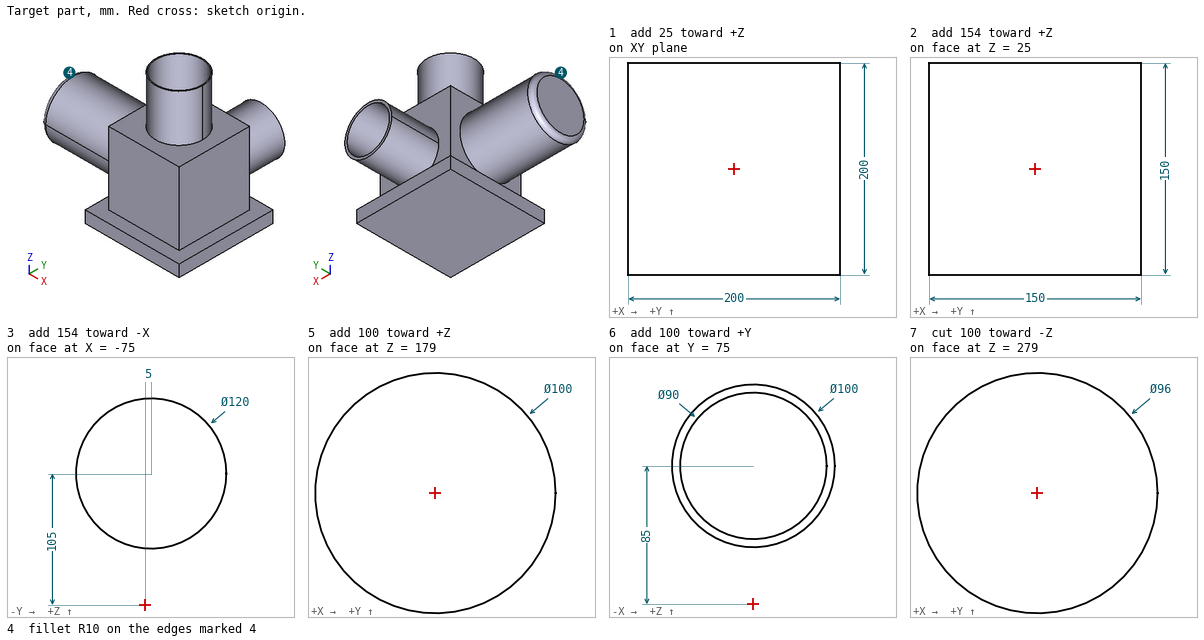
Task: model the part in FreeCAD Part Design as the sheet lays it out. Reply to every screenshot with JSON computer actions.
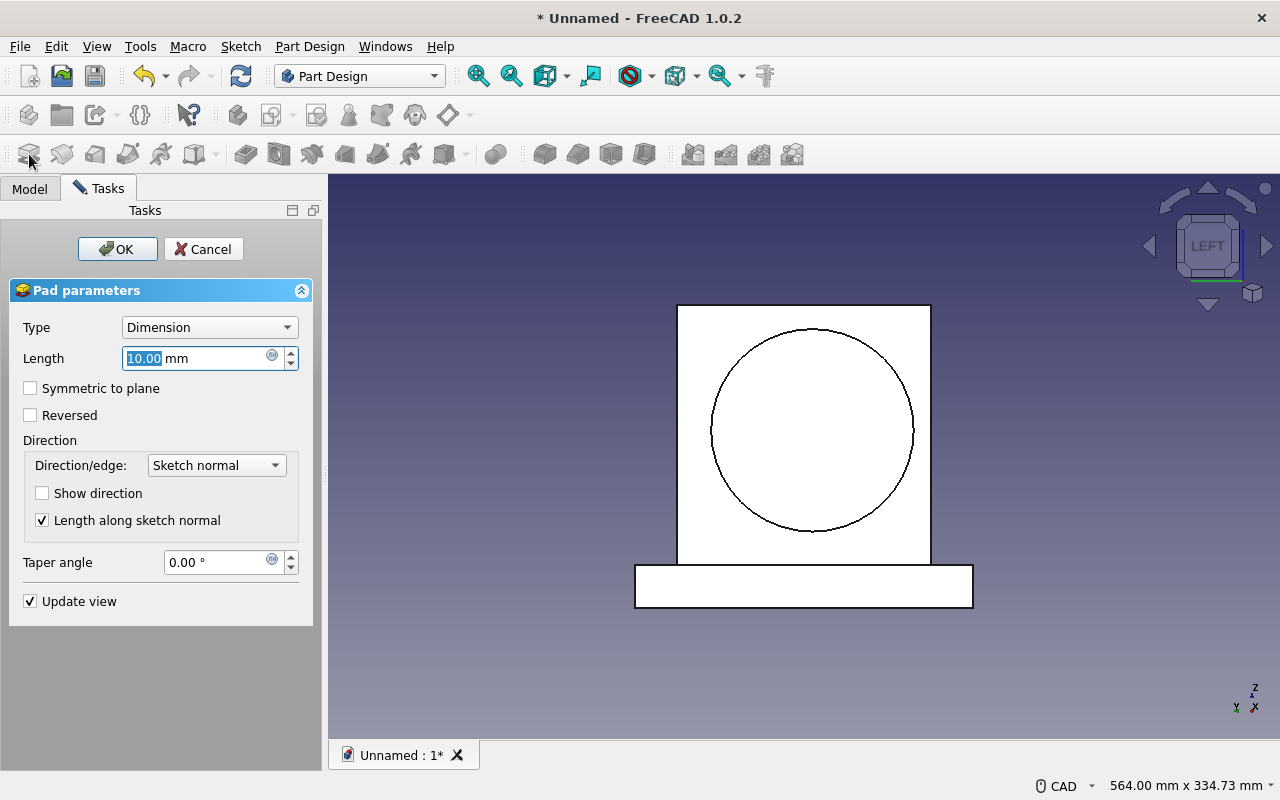
{"action": "type", "text": "154"}
{"action": "key", "text": "Tab"}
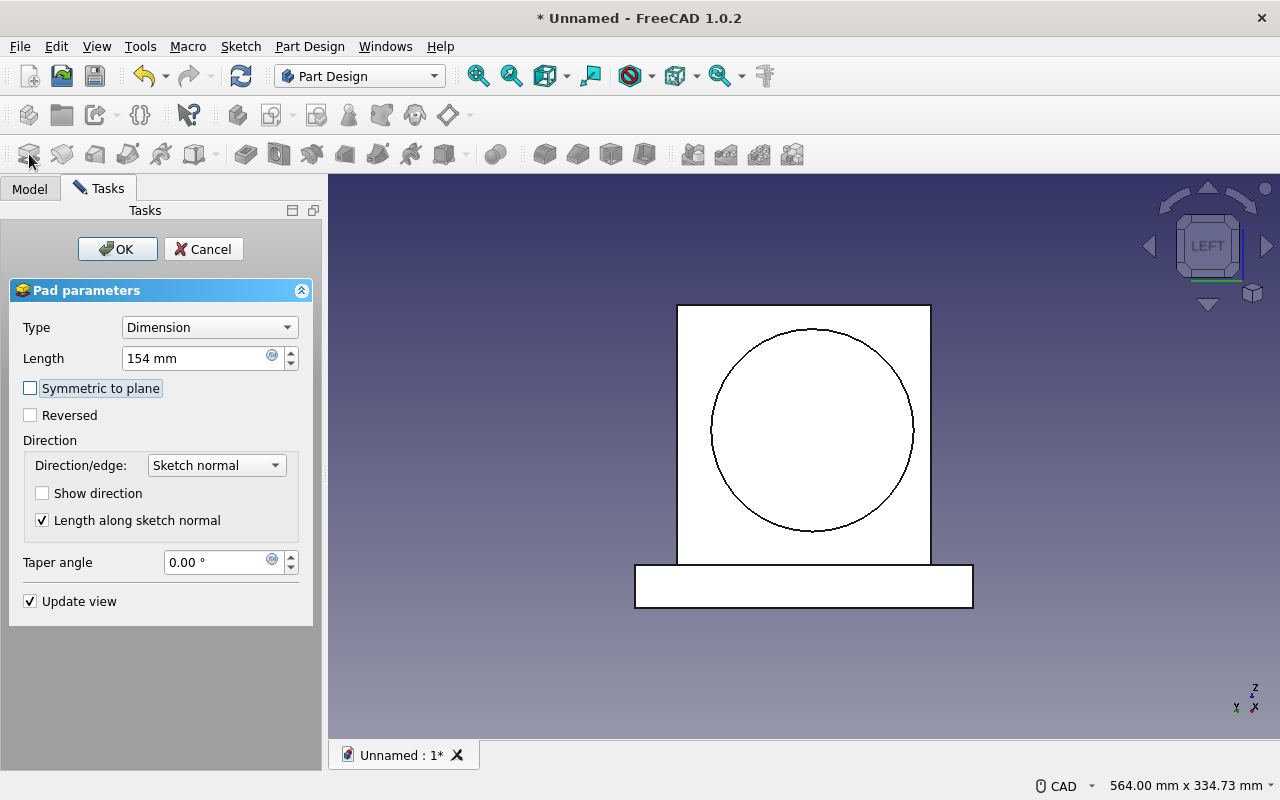
{"action": "left_click", "coordinate": [118, 249]}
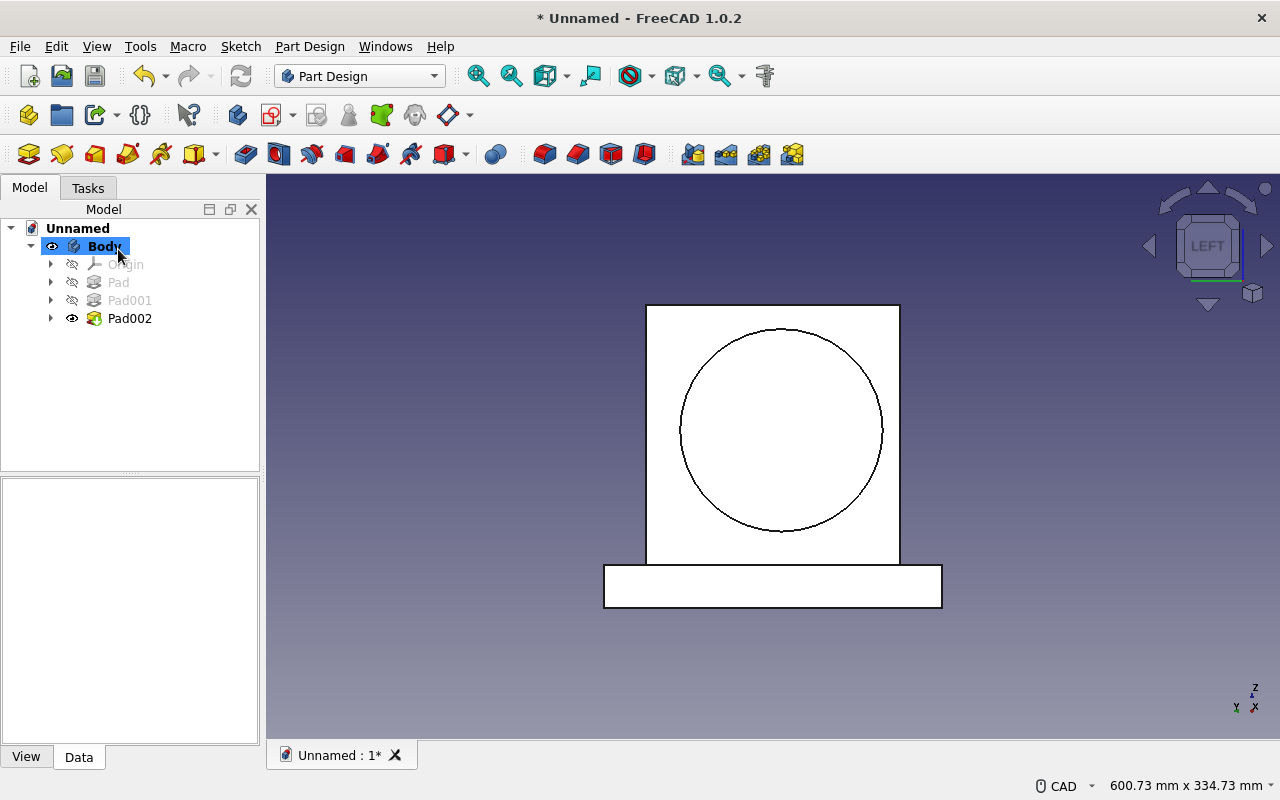
{"action": "left_click", "coordinate": [680, 429]}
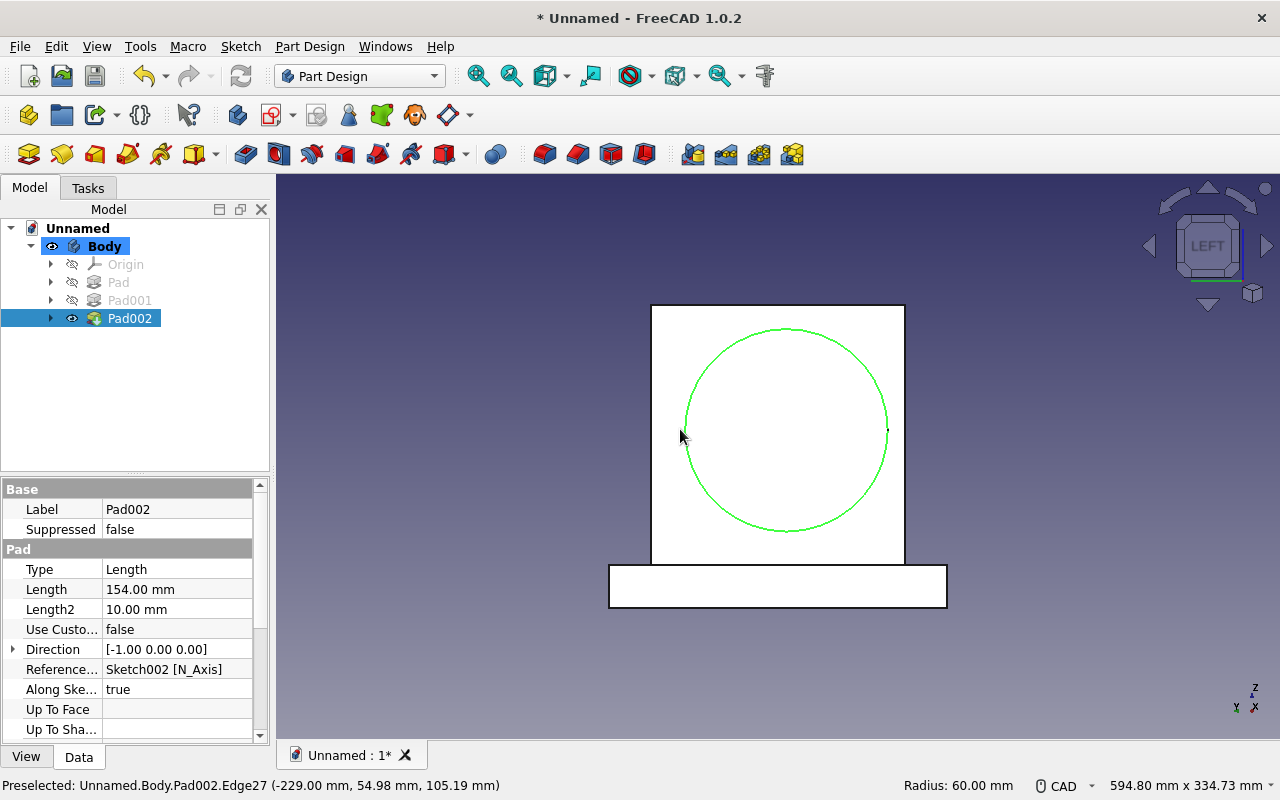
{"action": "left_click", "coordinate": [545, 154]}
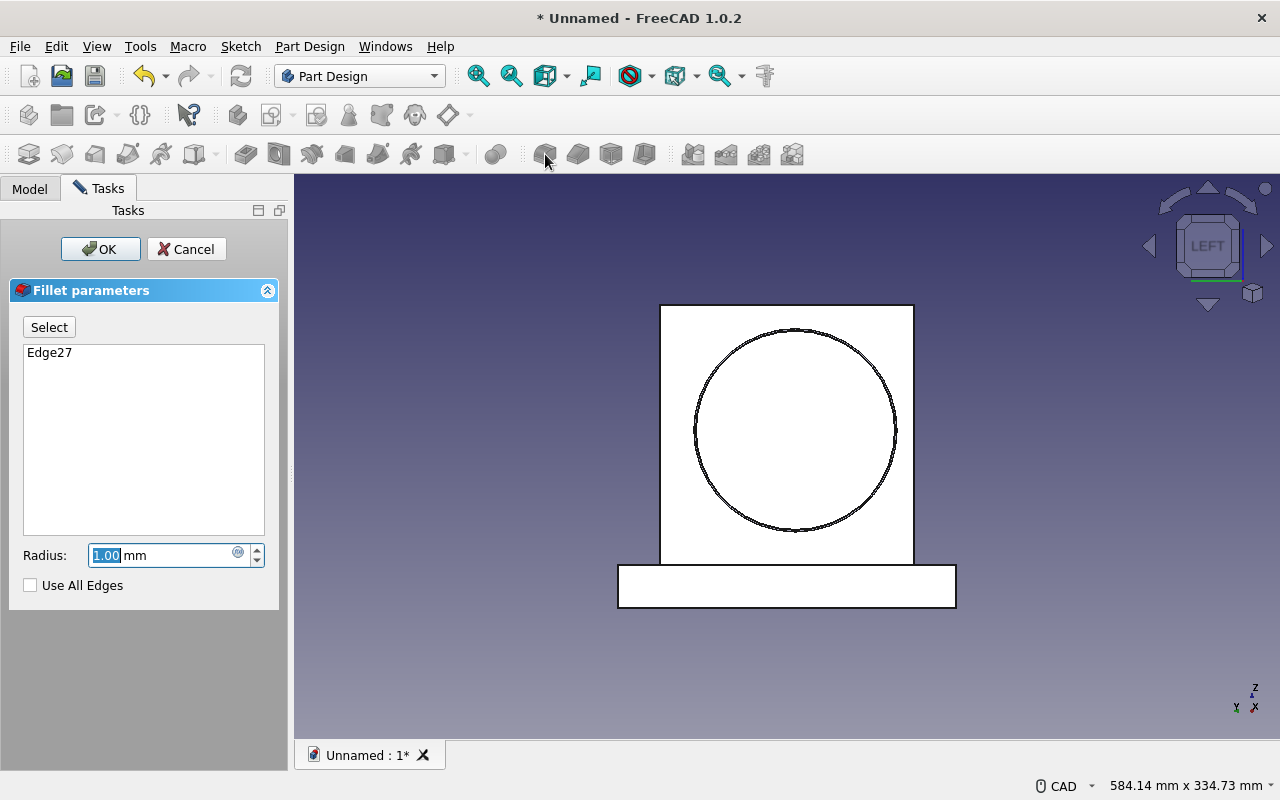
{"action": "type", "text": "10"}
{"action": "key", "text": "Tab"}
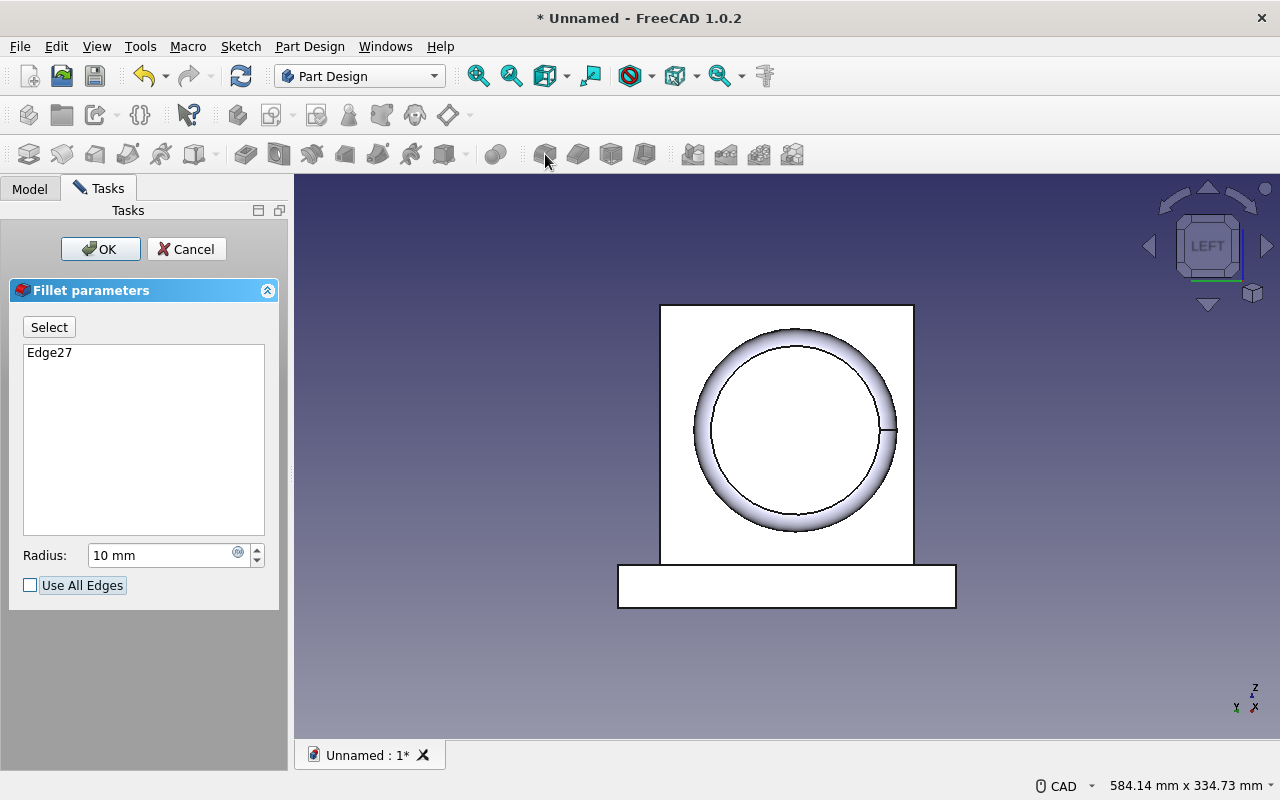
{"action": "left_click", "coordinate": [101, 249]}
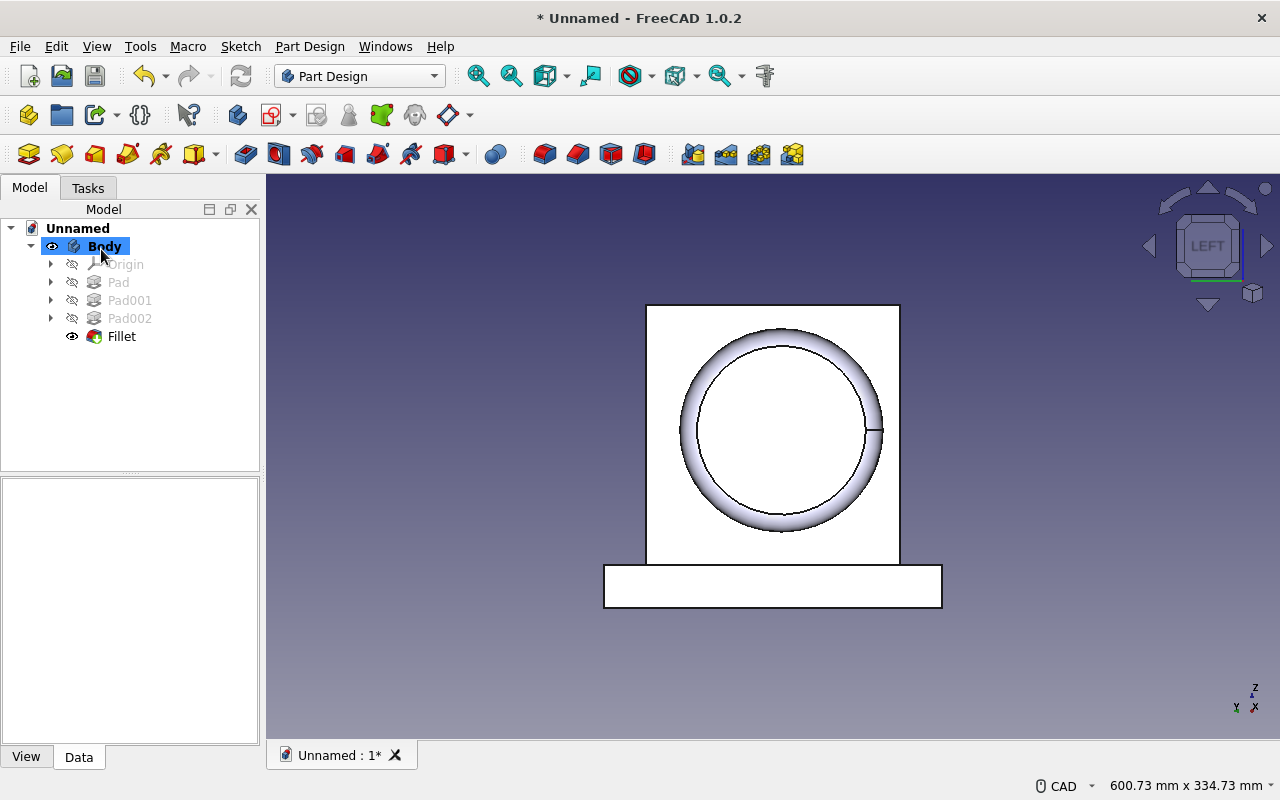
{"action": "key", "text": "0"}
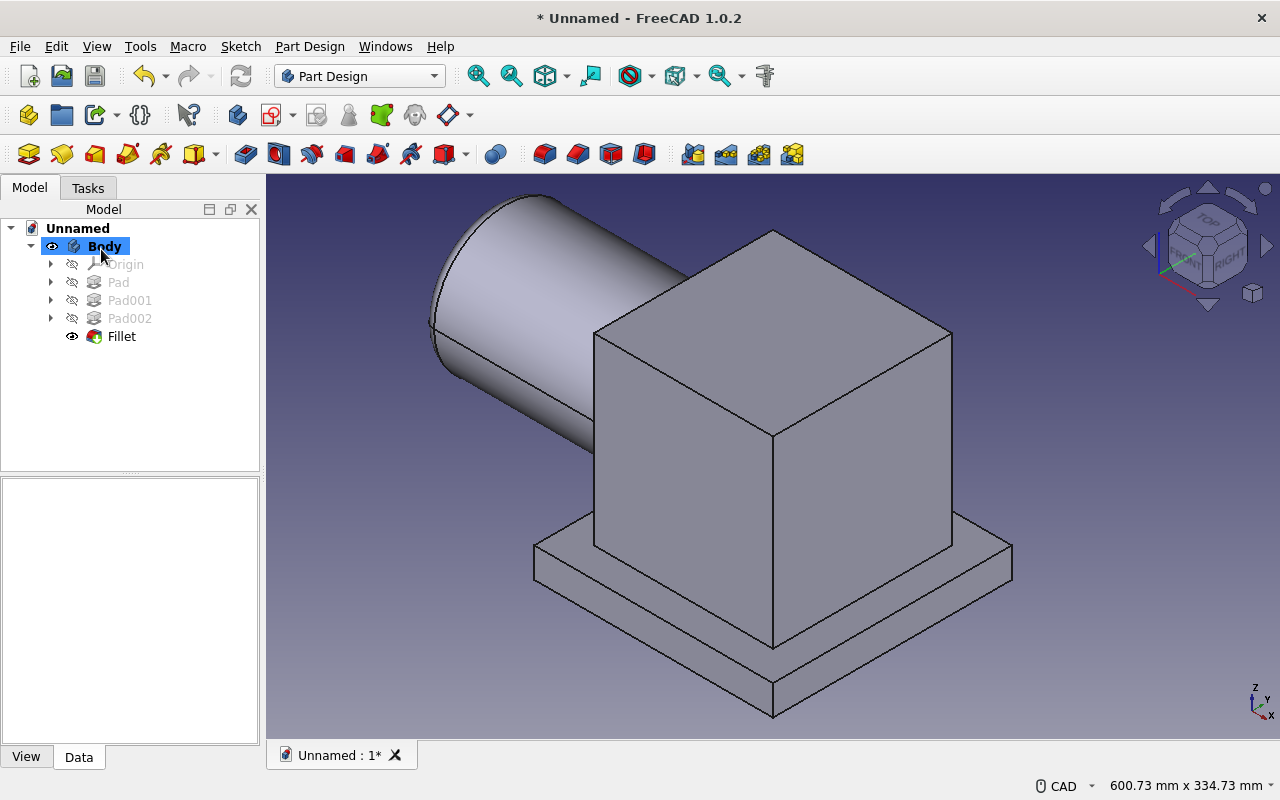
{"action": "left_click", "coordinate": [479, 76]}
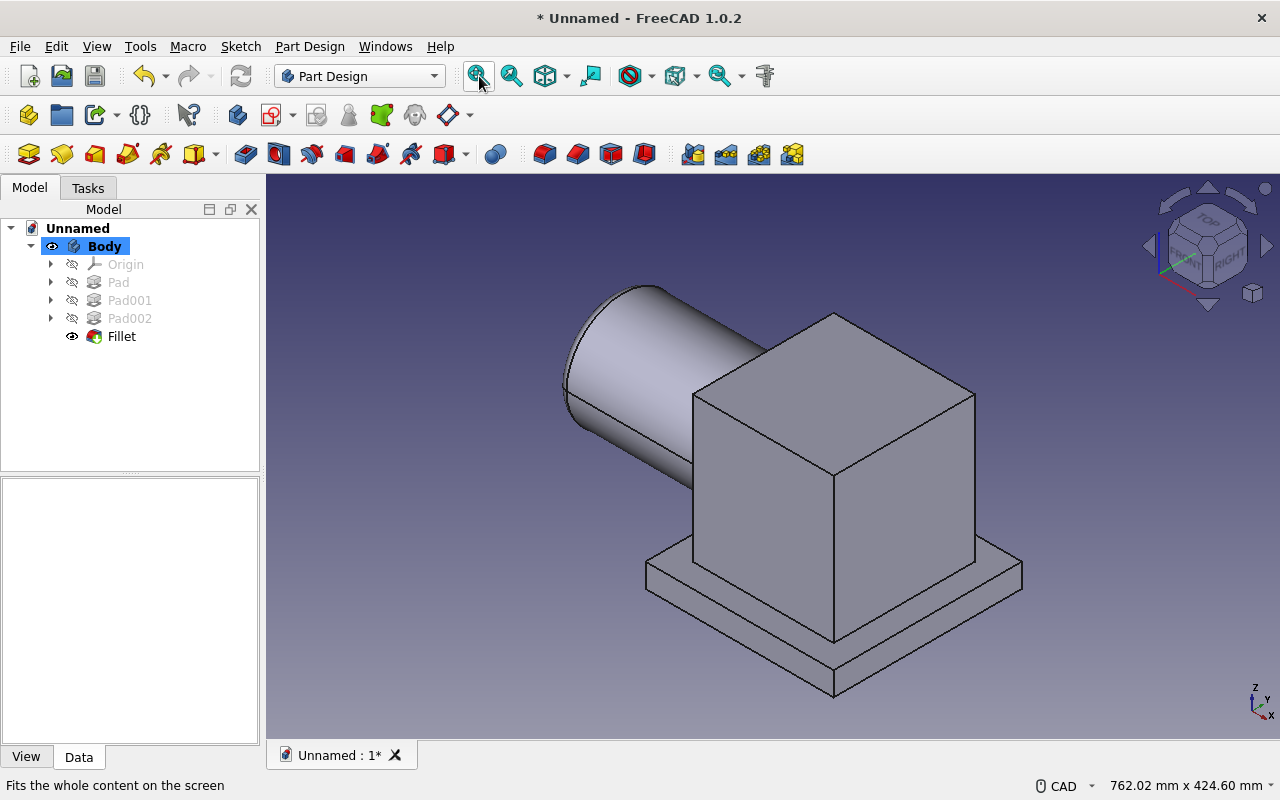
{"action": "left_click", "coordinate": [834, 393]}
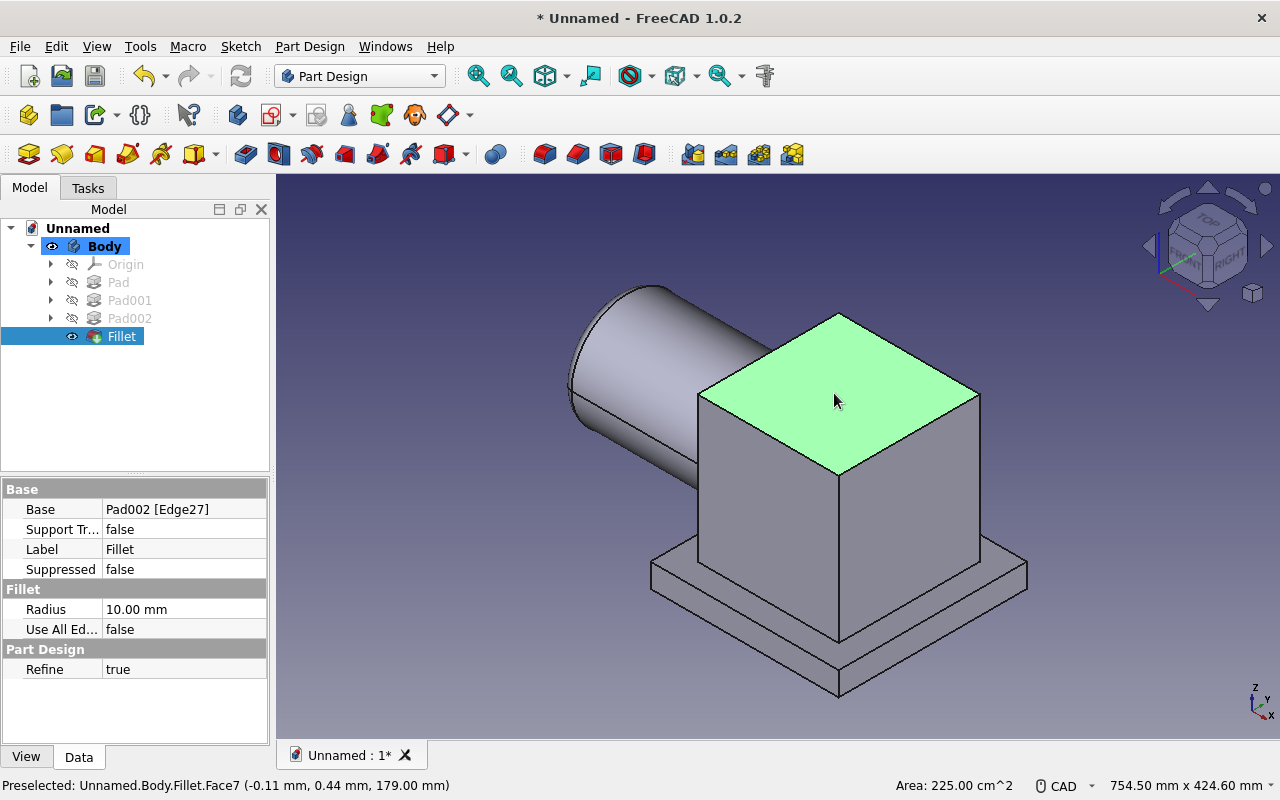
{"action": "left_click", "coordinate": [270, 116]}